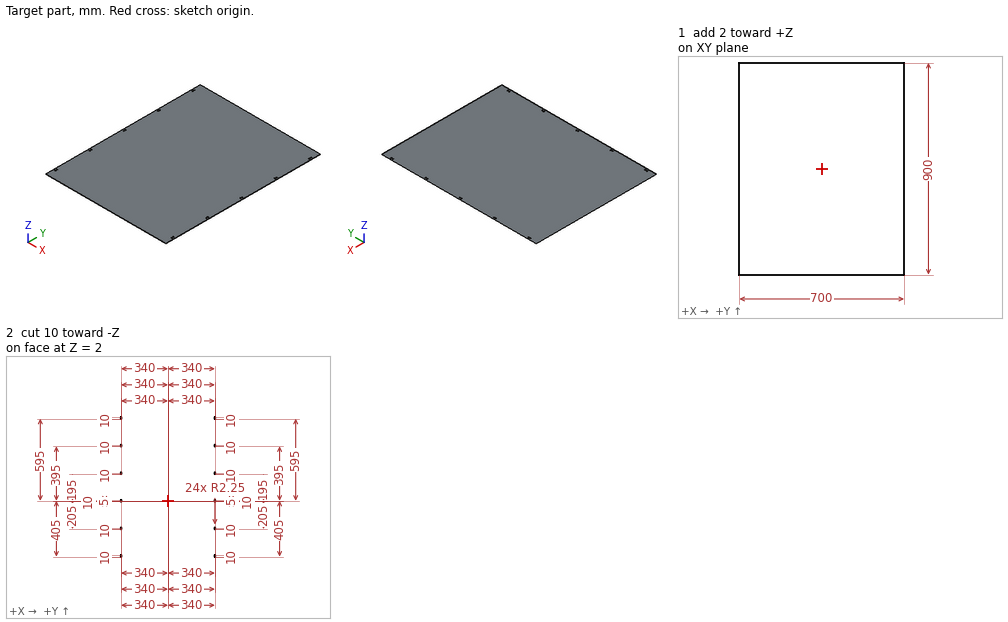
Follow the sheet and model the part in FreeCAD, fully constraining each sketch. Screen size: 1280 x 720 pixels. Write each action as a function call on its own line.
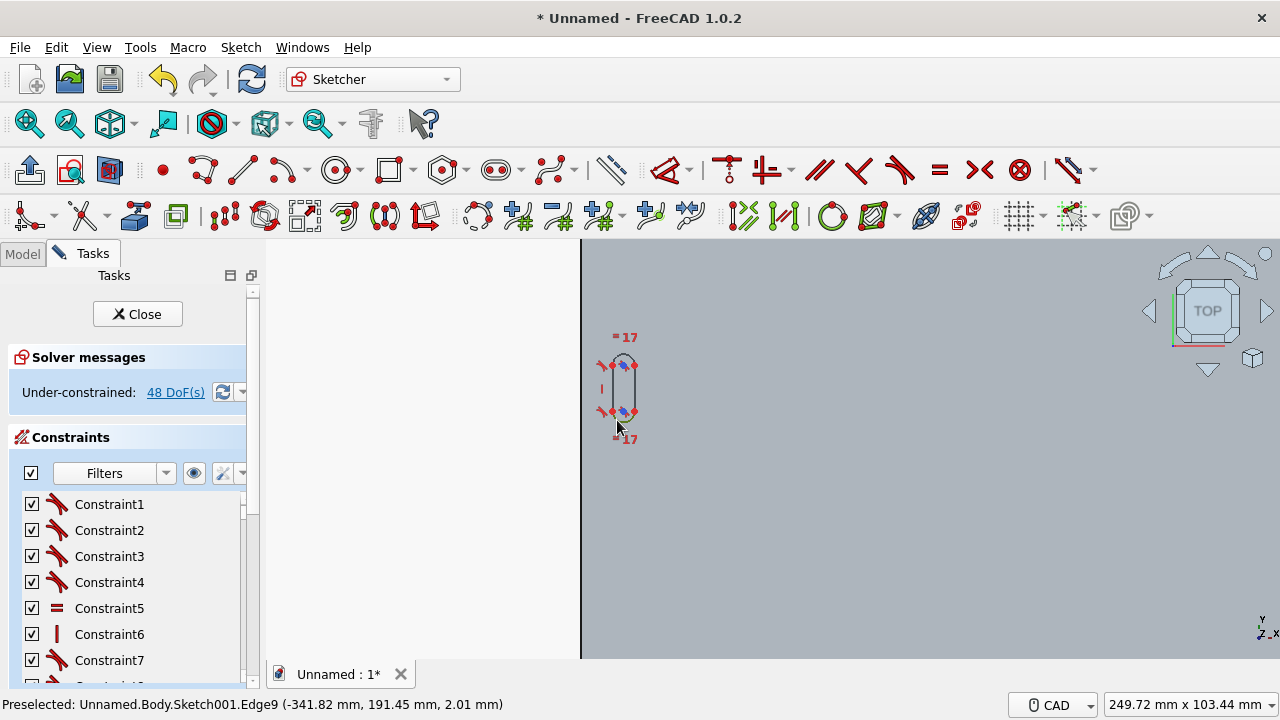
scroll(620, 427, down, 14)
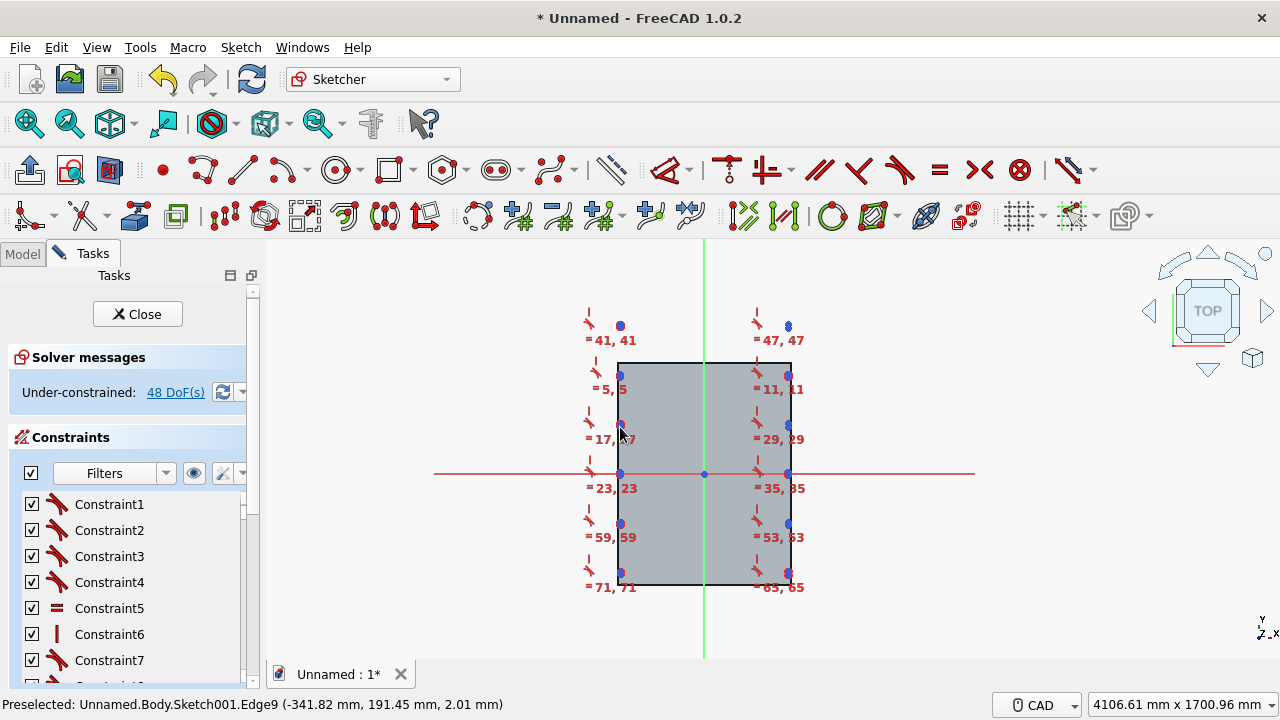
scroll(620, 476, up, 14)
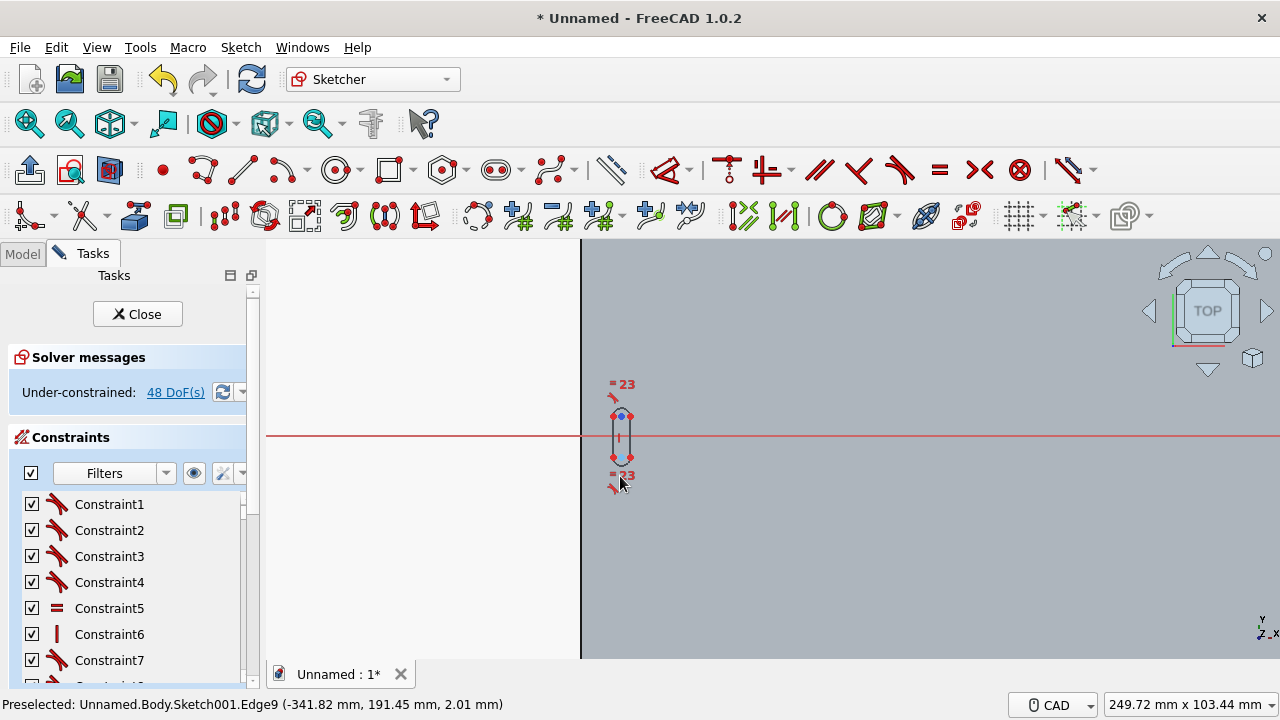
click(622, 466)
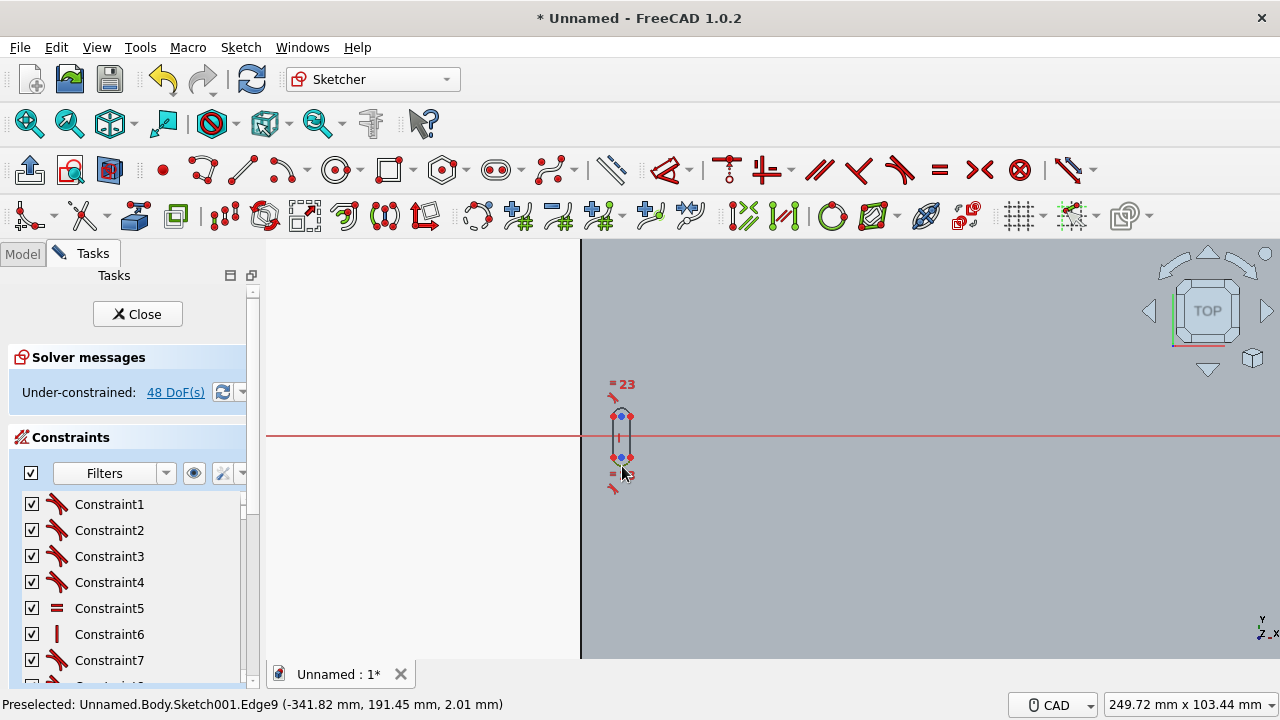
scroll(620, 476, down, 14)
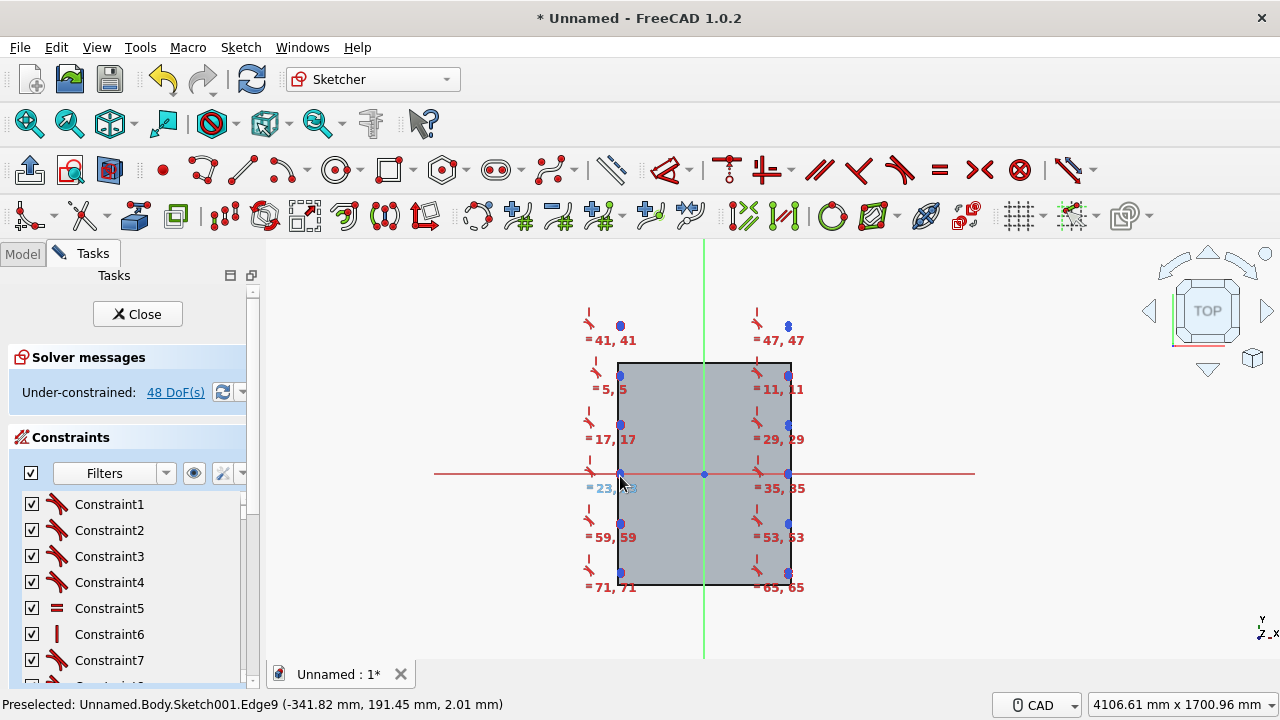
scroll(789, 427, up, 14)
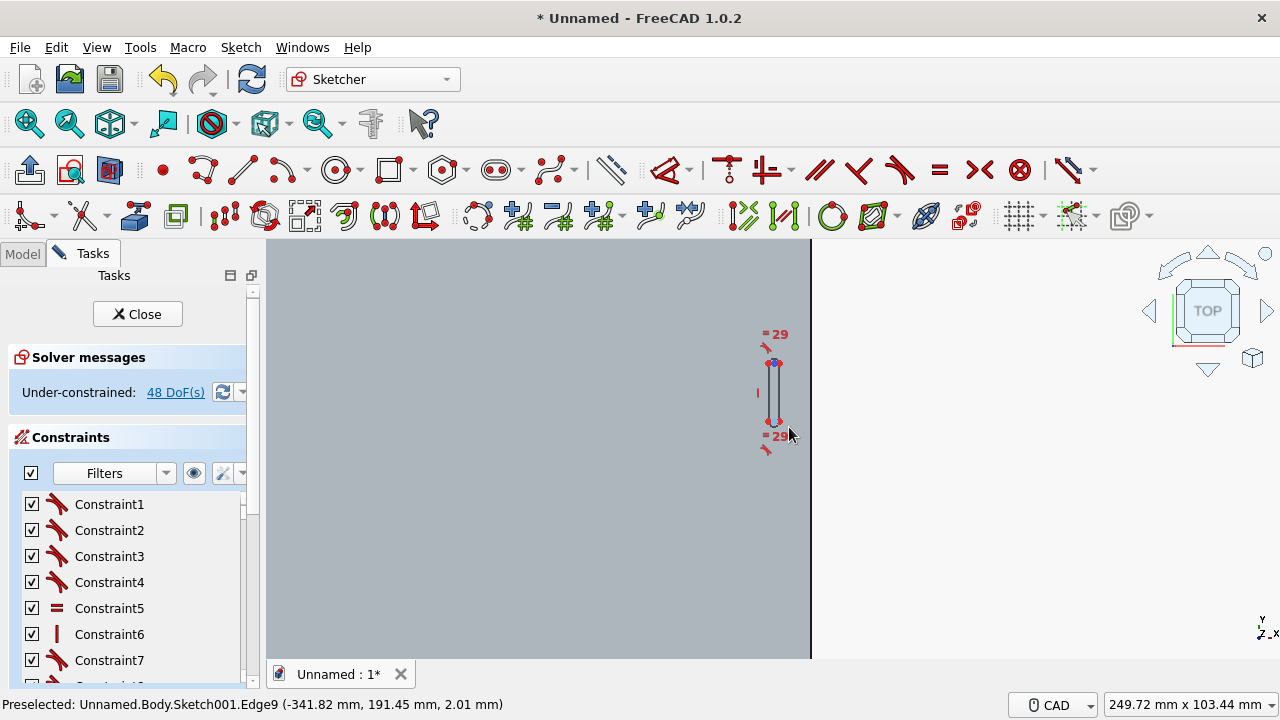
click(774, 427)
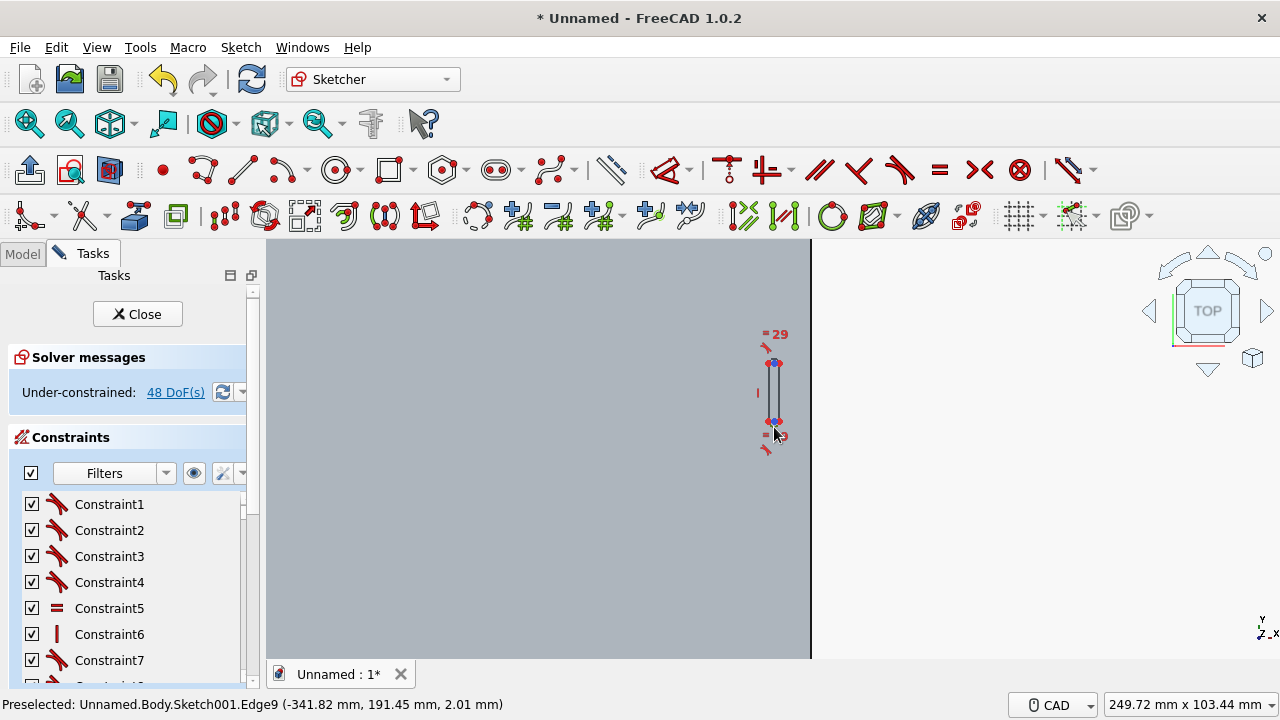
scroll(790, 427, down, 14)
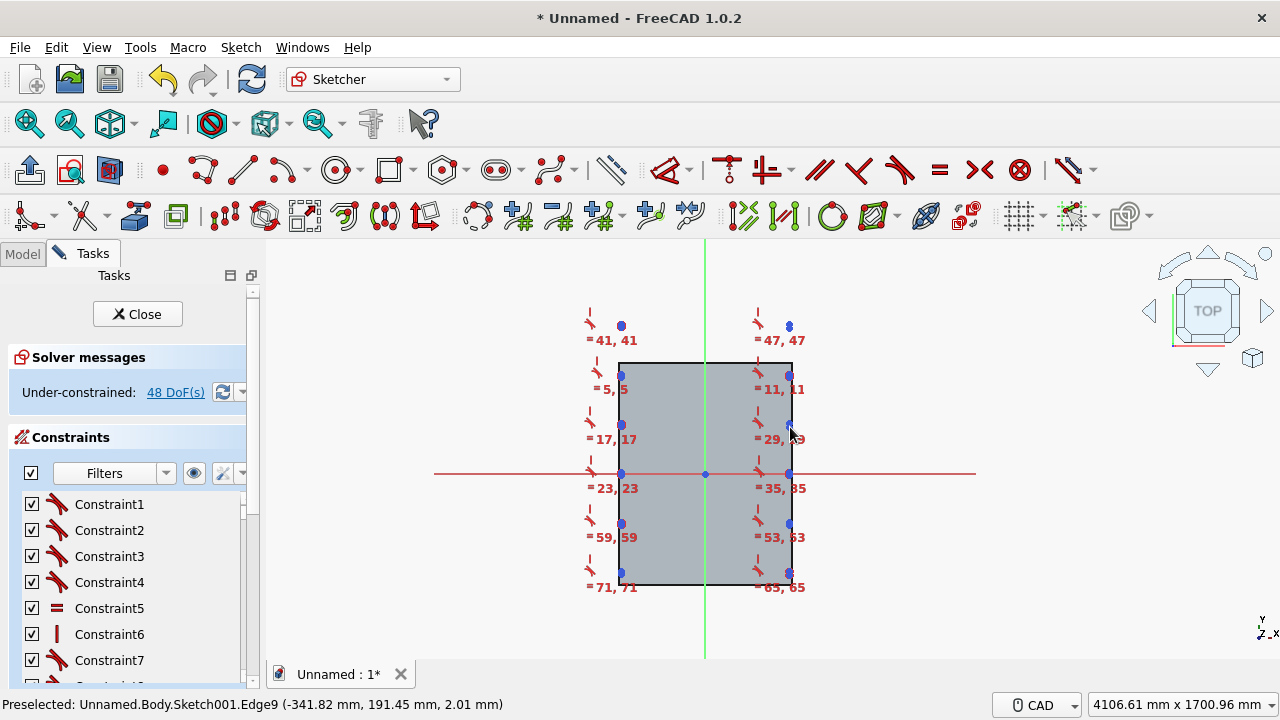
scroll(789, 476, up, 14)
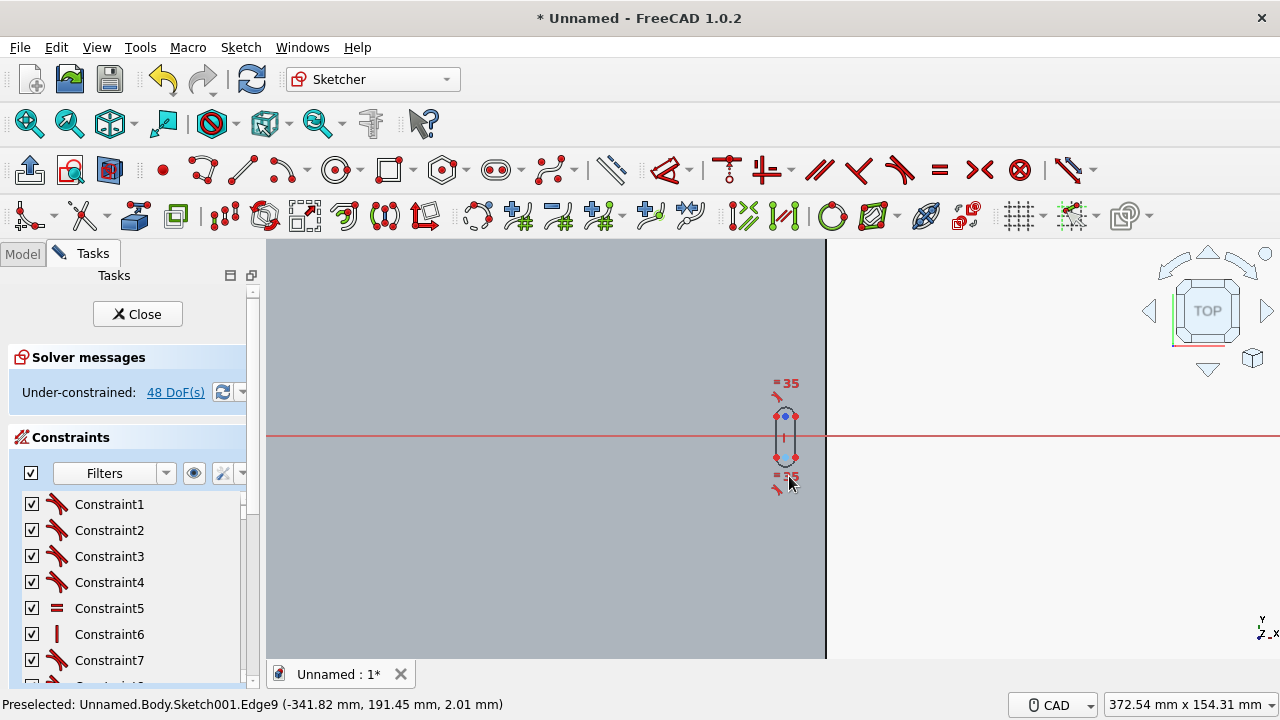
click(786, 467)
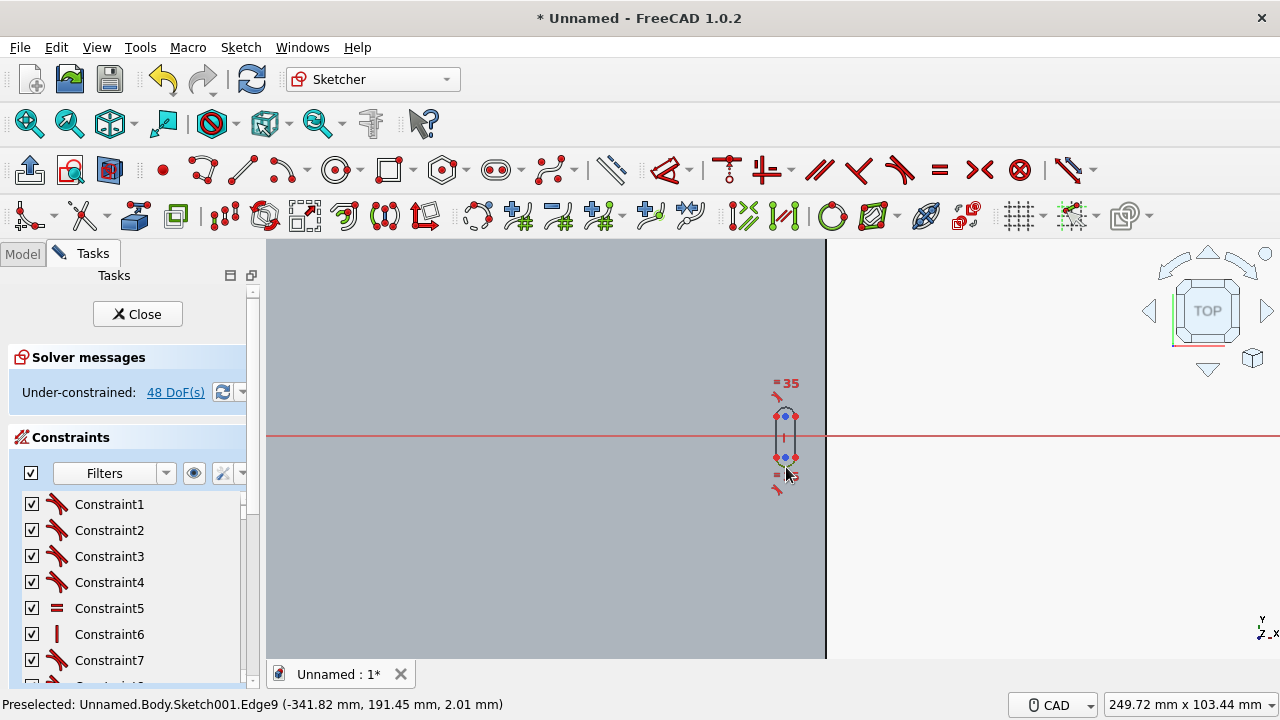
scroll(789, 476, down, 14)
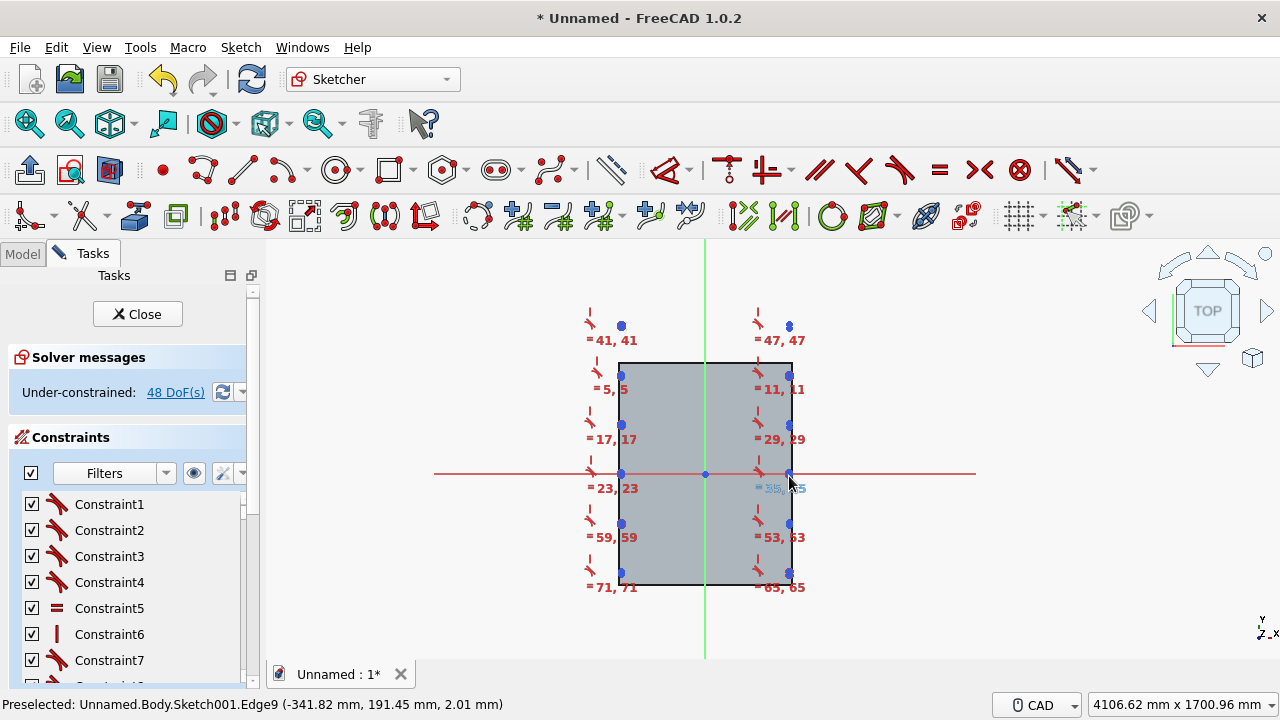
scroll(621, 328, up, 14)